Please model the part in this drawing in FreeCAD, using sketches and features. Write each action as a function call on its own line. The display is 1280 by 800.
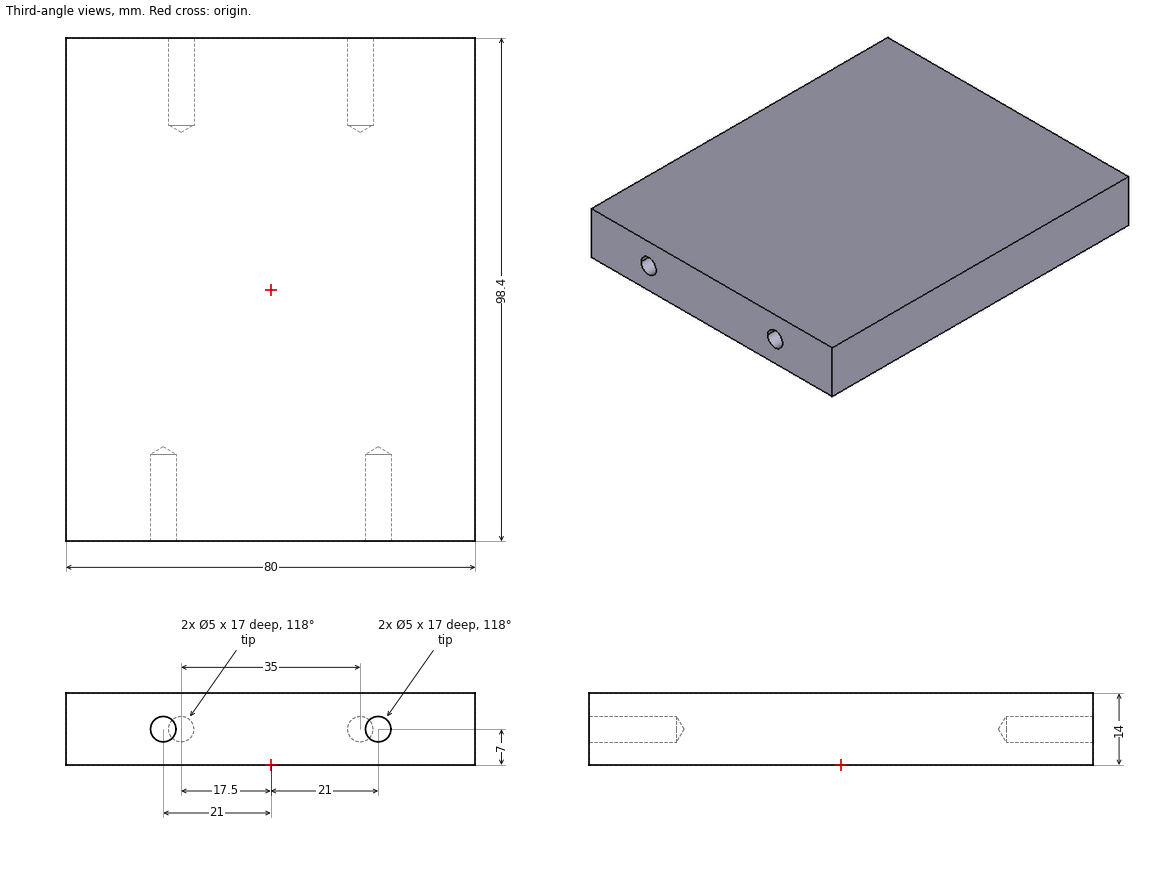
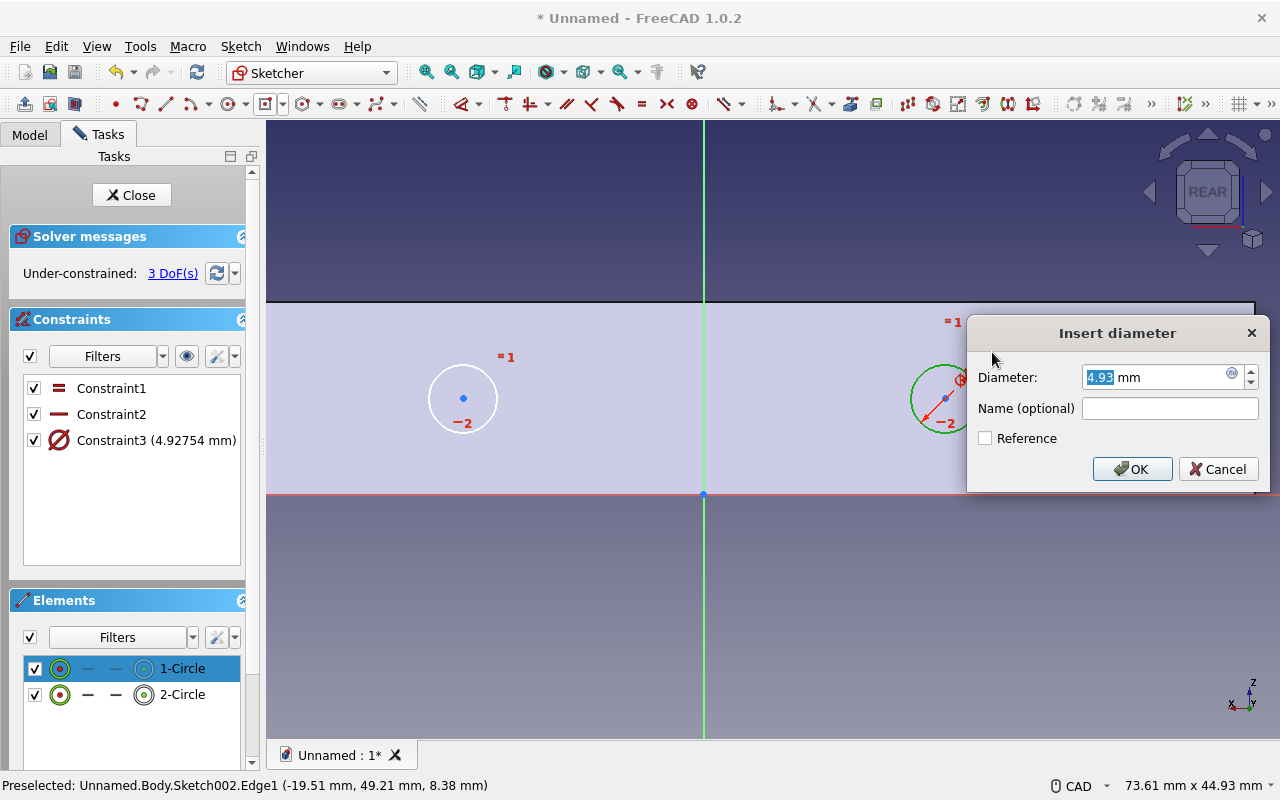
text(5)
key(Return)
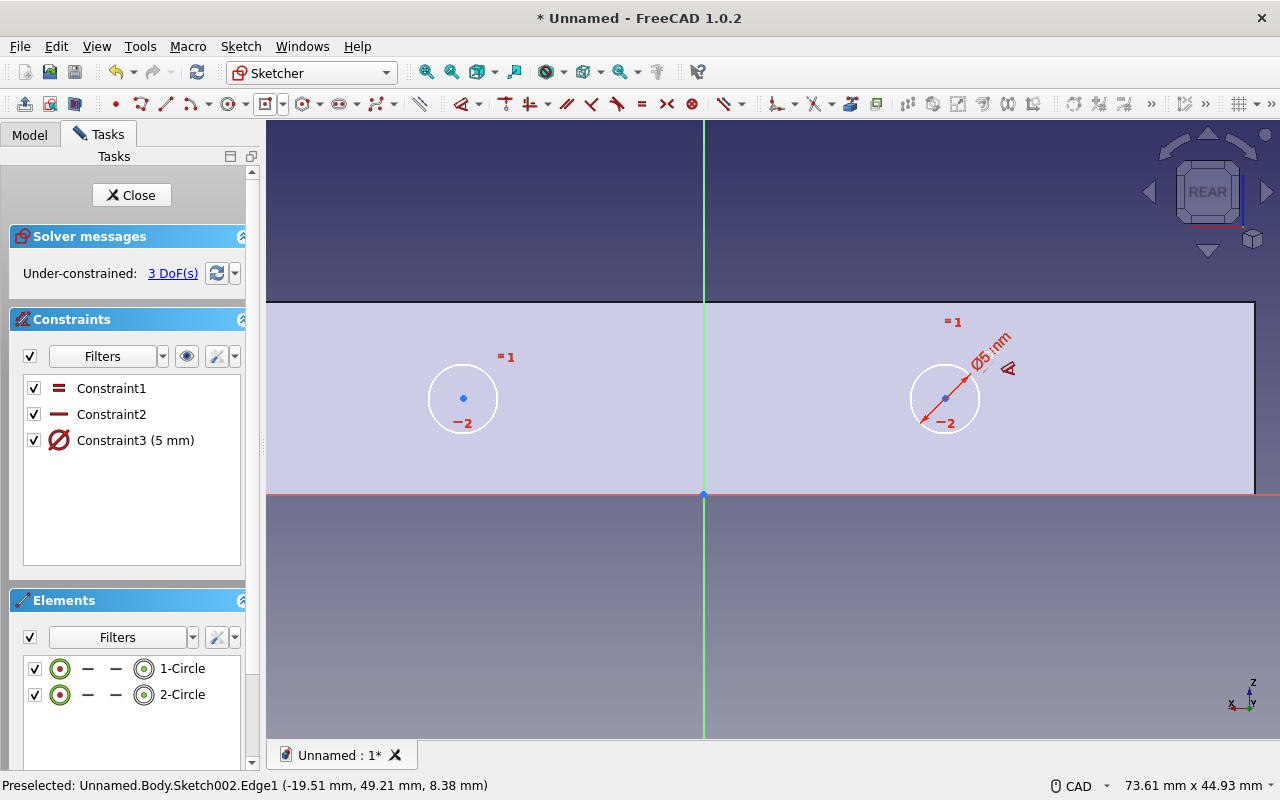
click(945, 399)
click(979, 447)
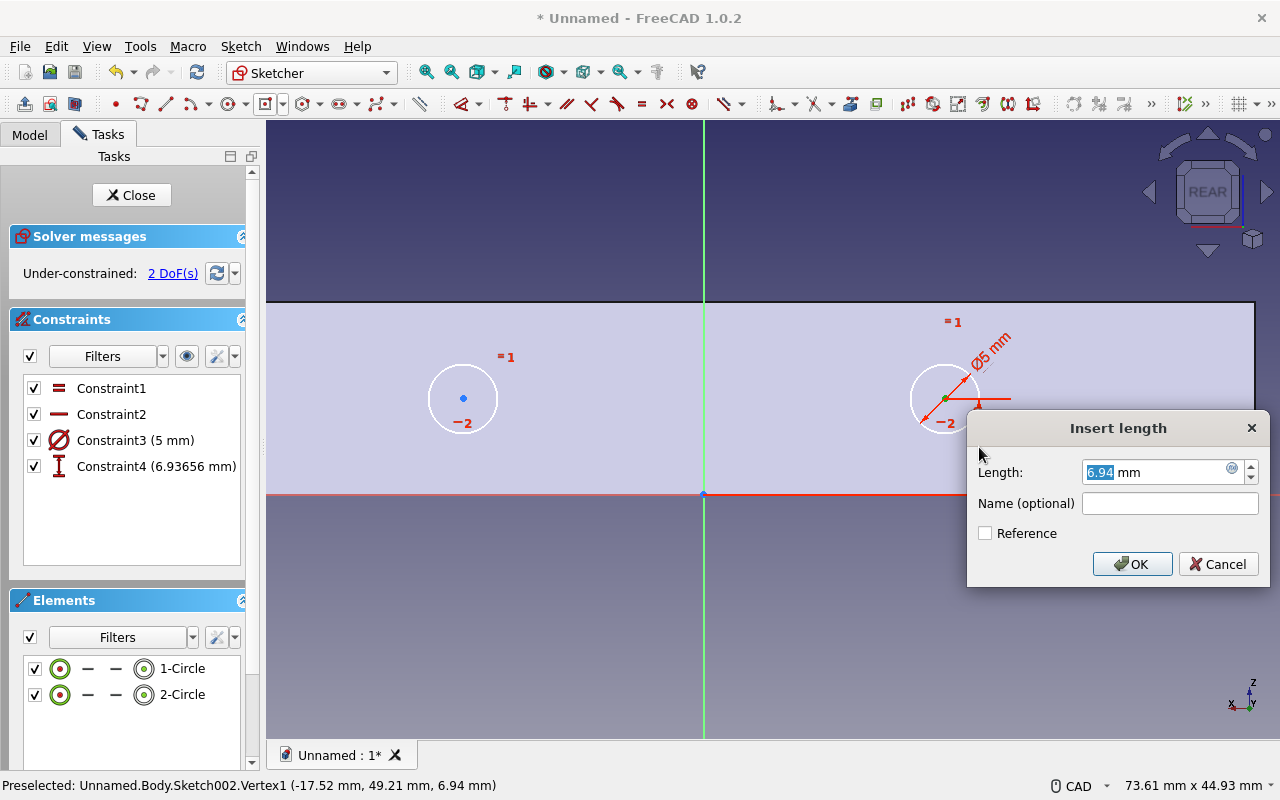
text(7)
key(Return)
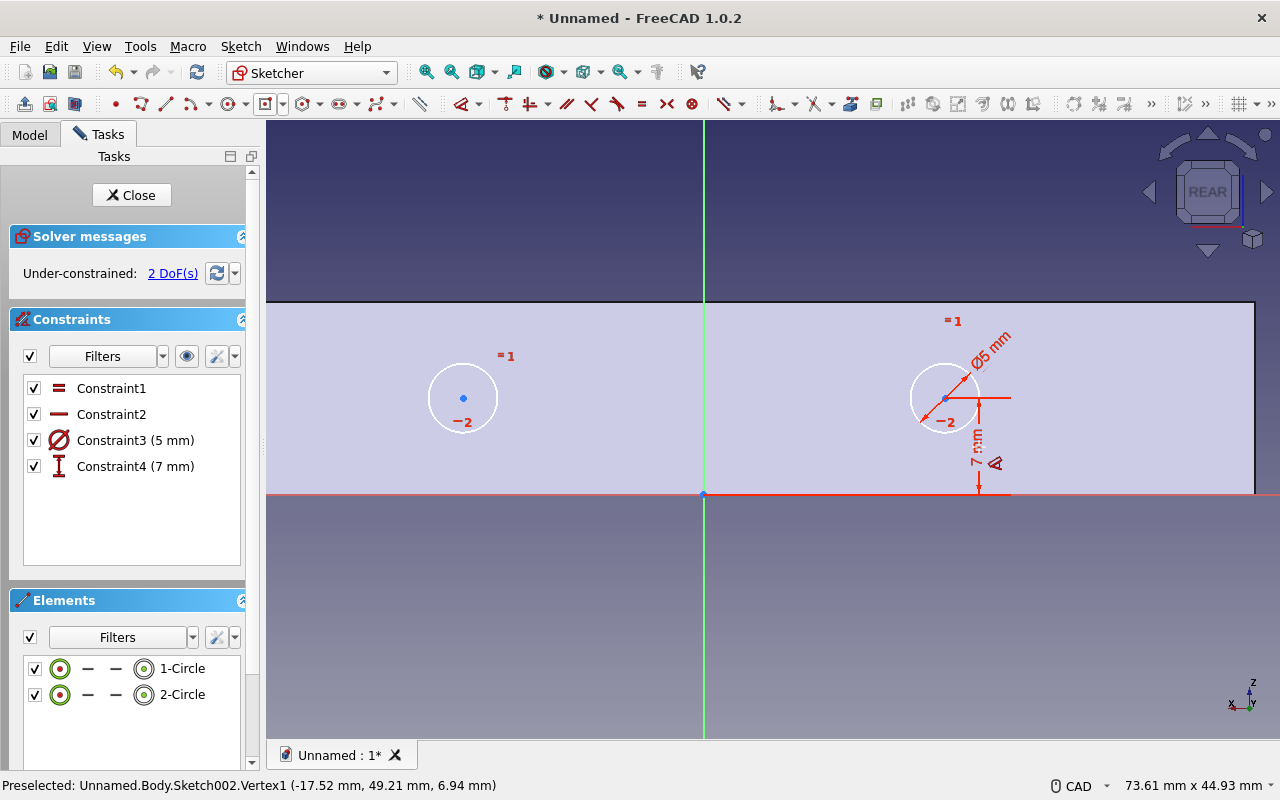
click(945, 398)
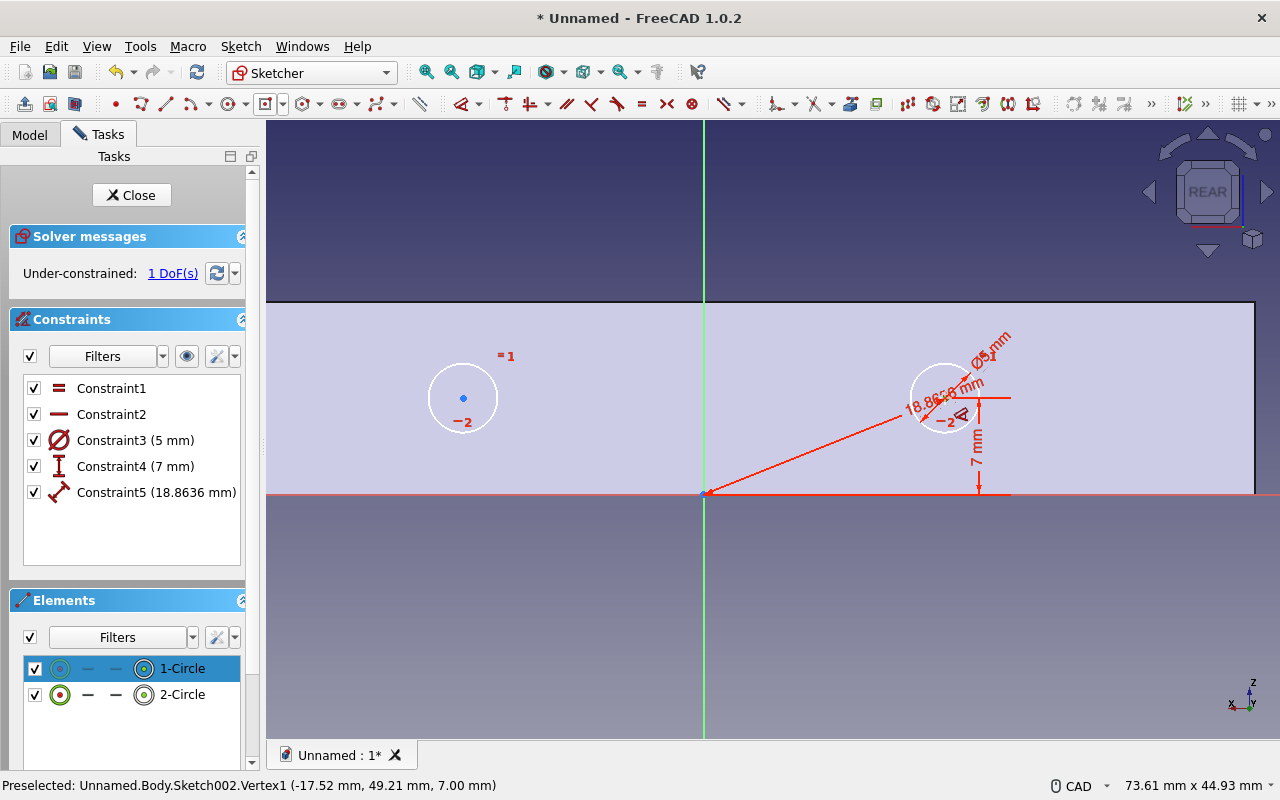
click(463, 398)
click(593, 364)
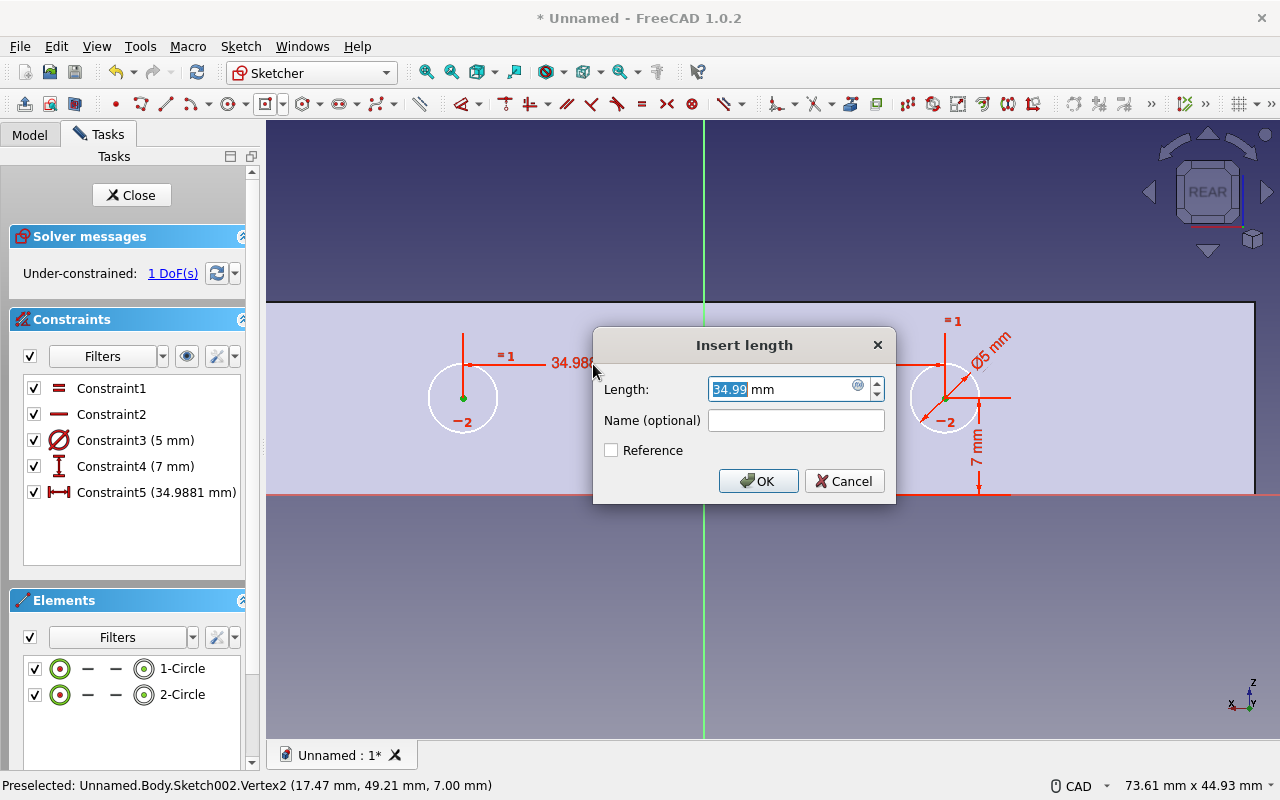
text(35)
key(Return)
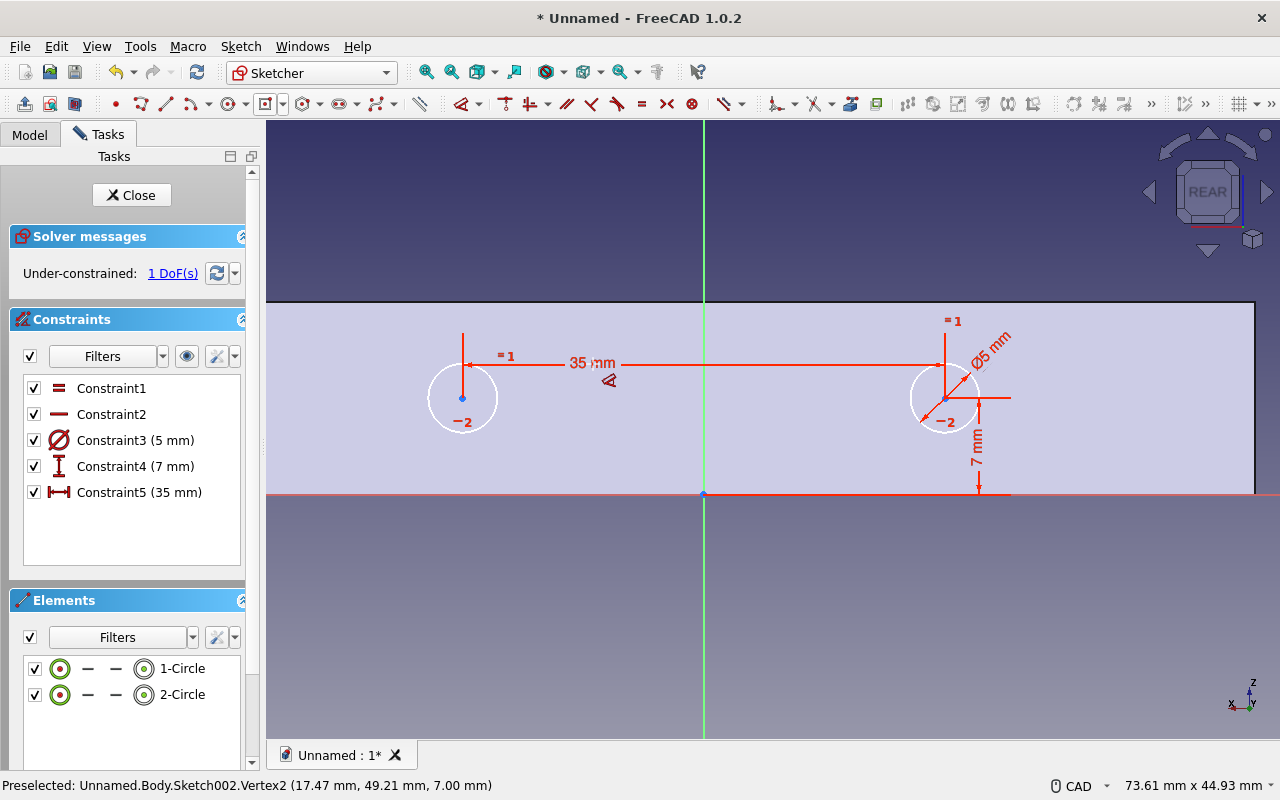
click(945, 398)
click(824, 529)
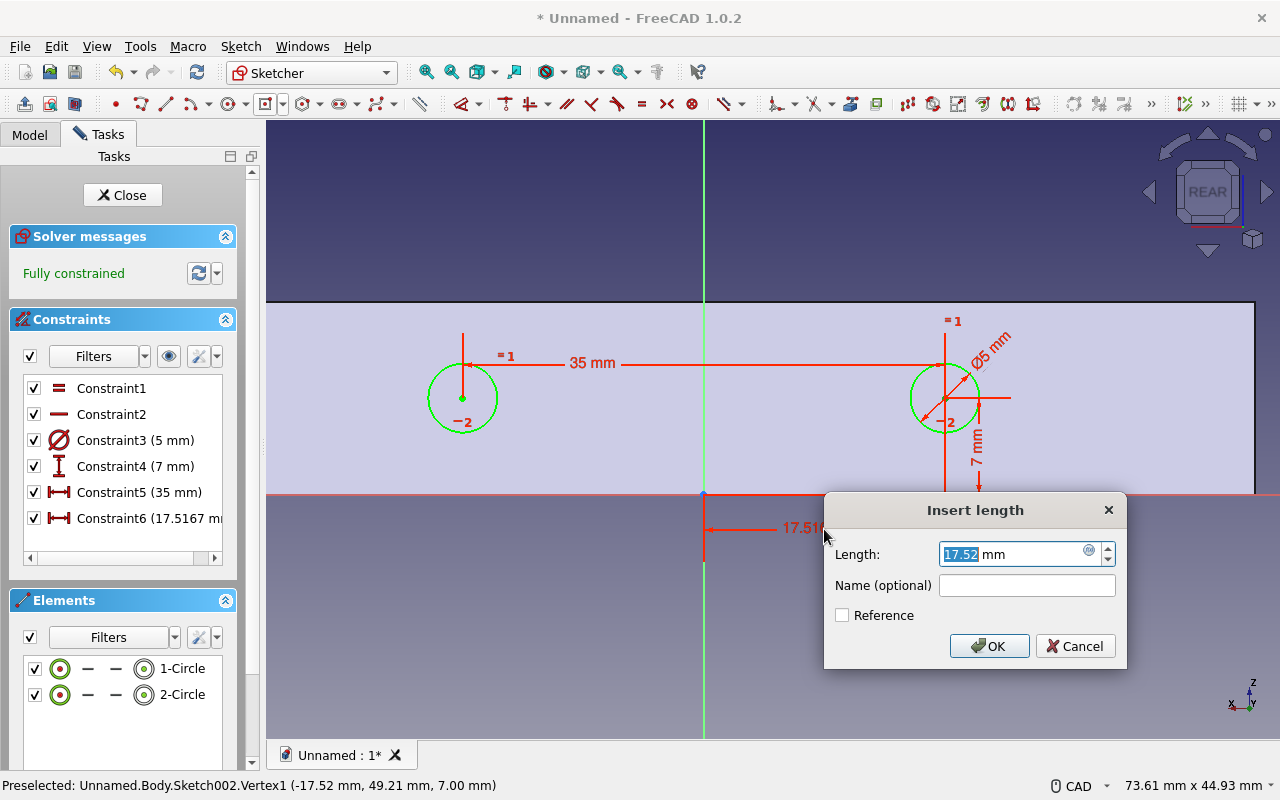
text(17.5)
key(Return)
key(Escape)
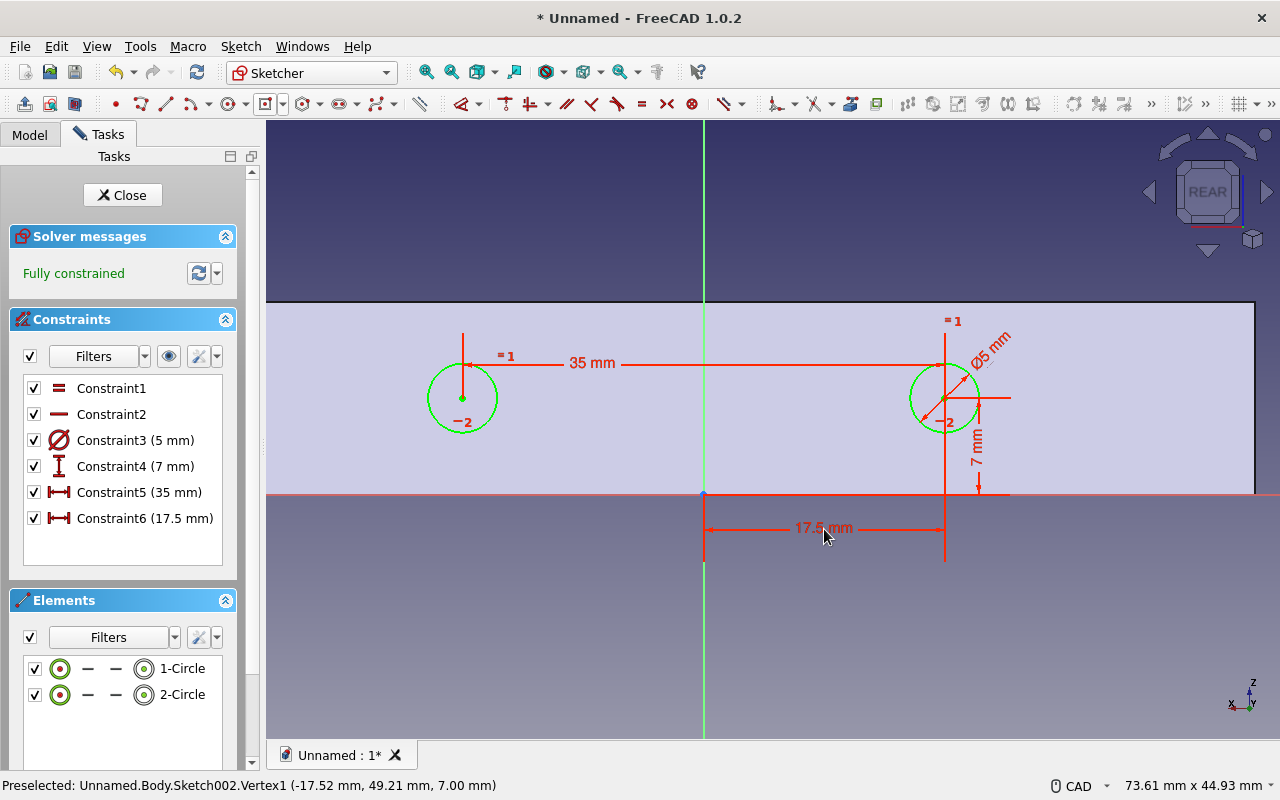
click(123, 195)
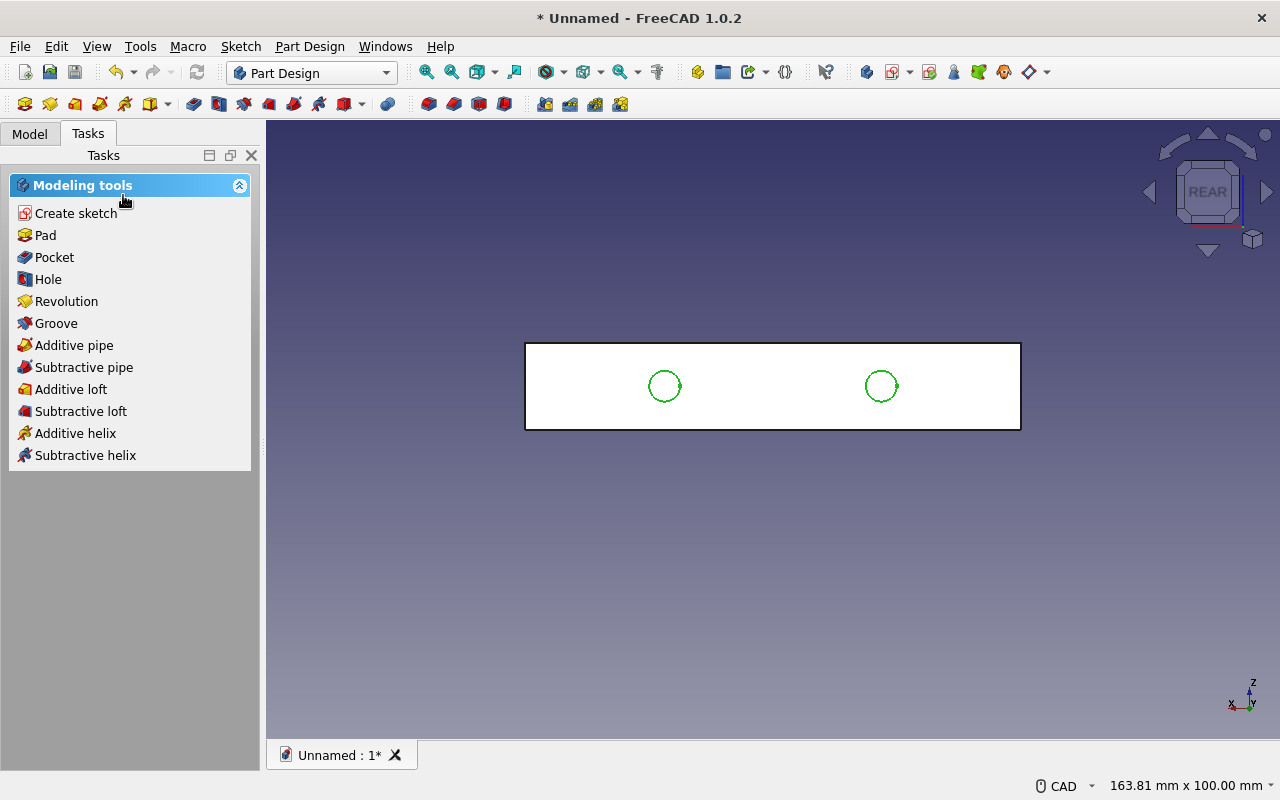
click(219, 104)